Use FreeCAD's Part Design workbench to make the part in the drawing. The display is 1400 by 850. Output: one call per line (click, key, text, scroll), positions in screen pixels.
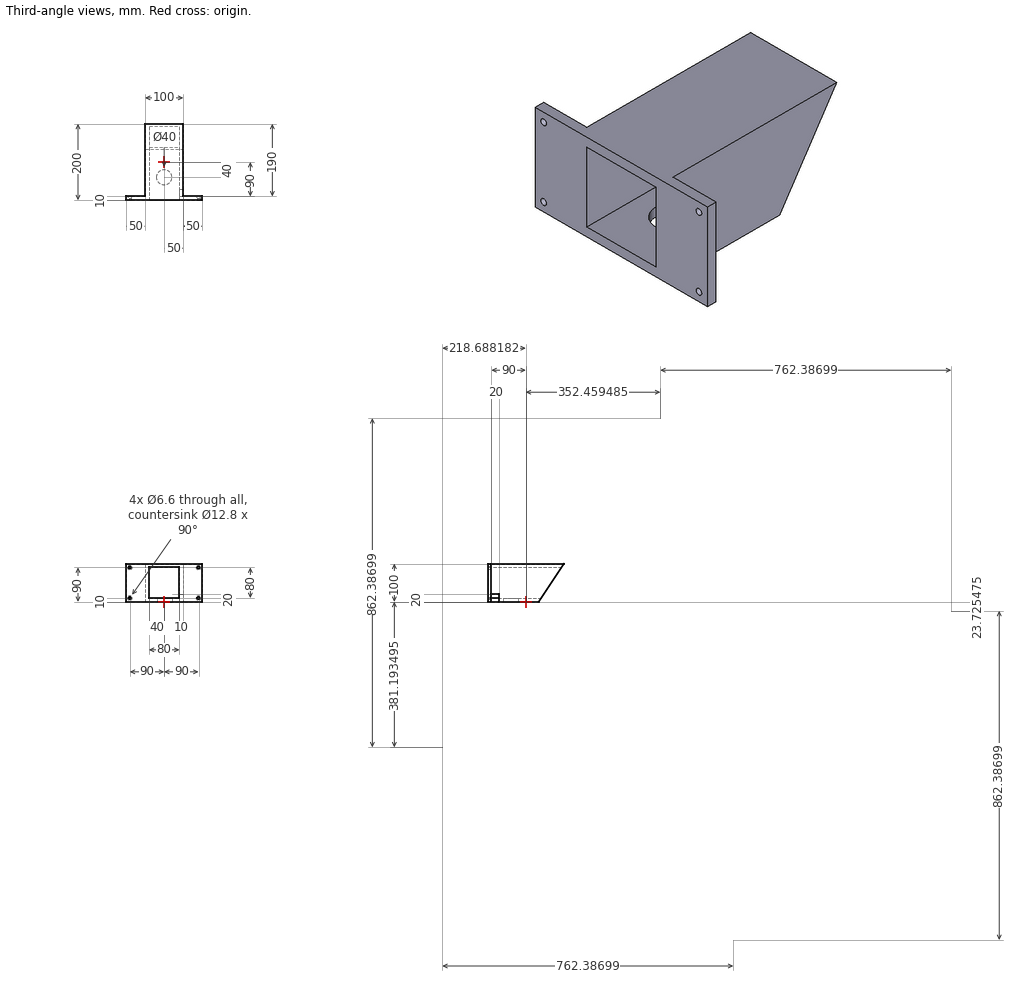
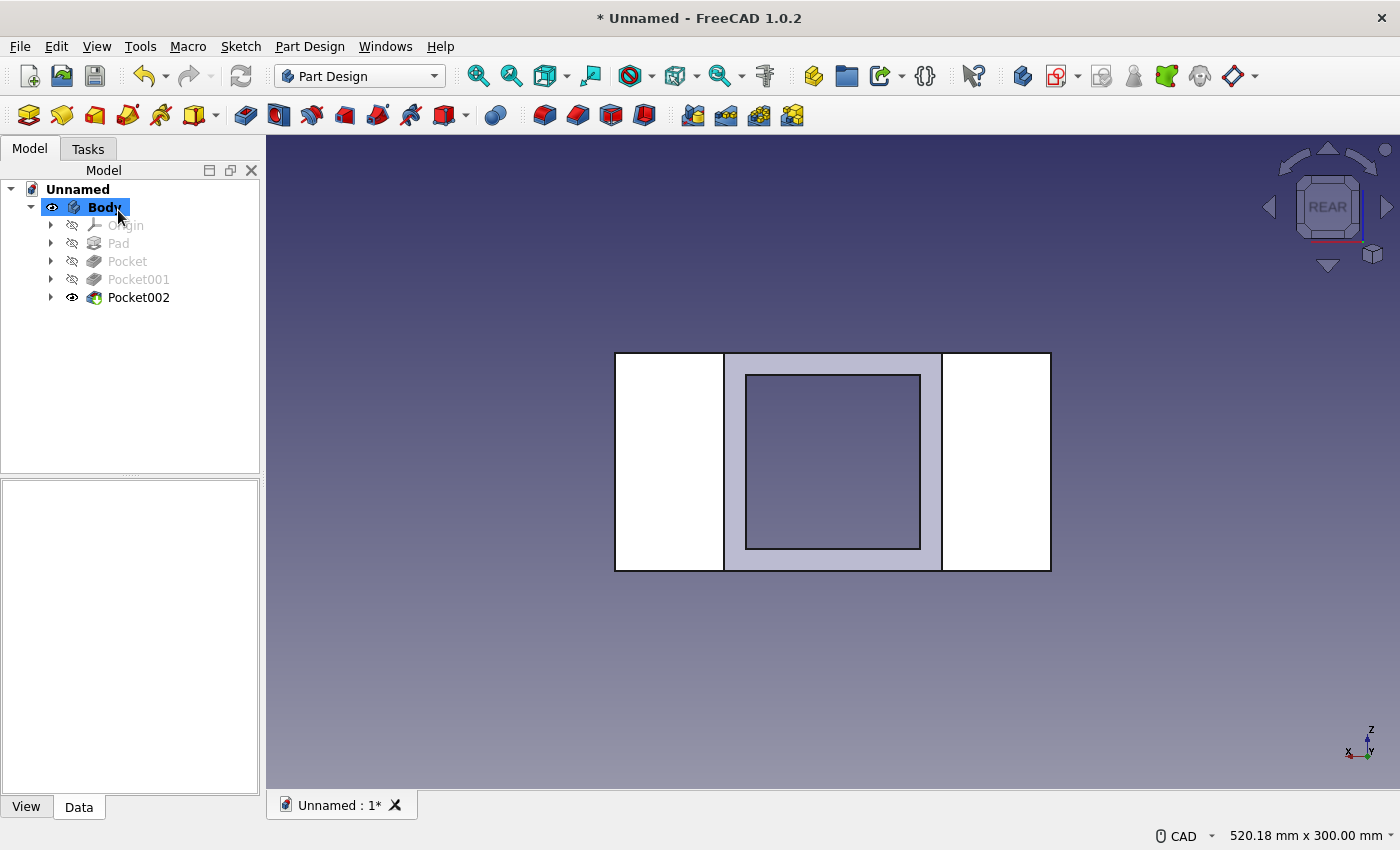
click(670, 430)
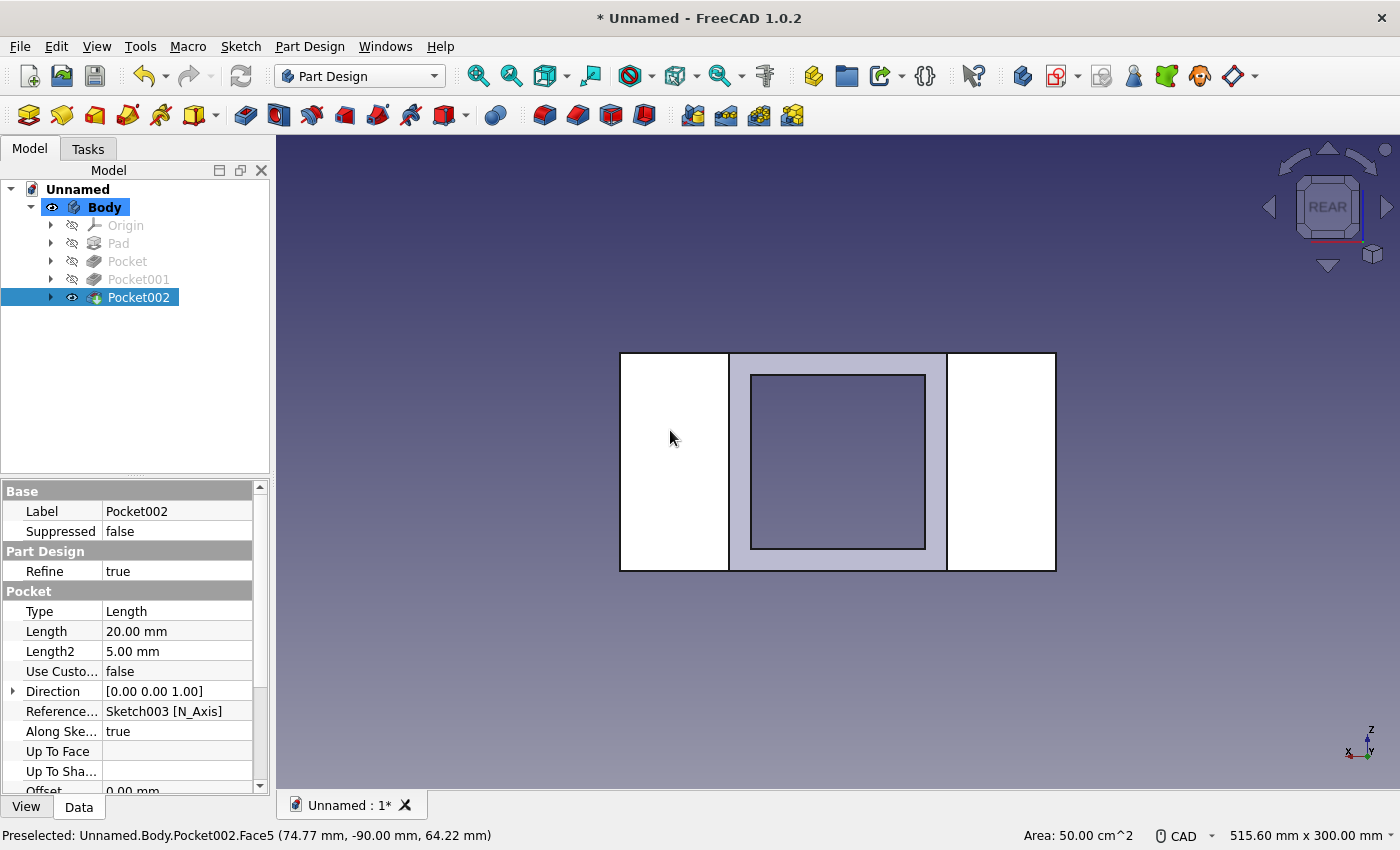
click(1056, 76)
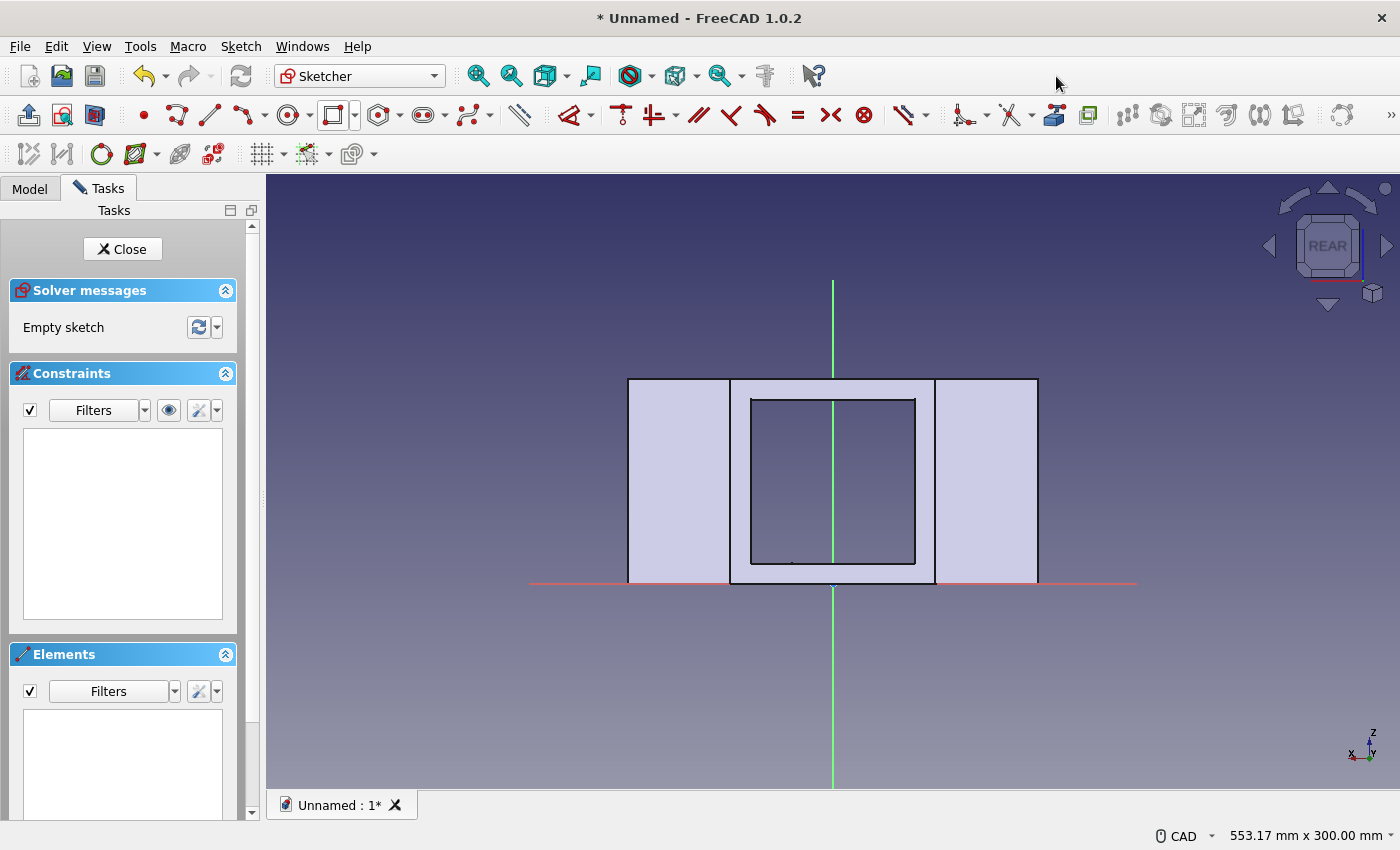
click(95, 116)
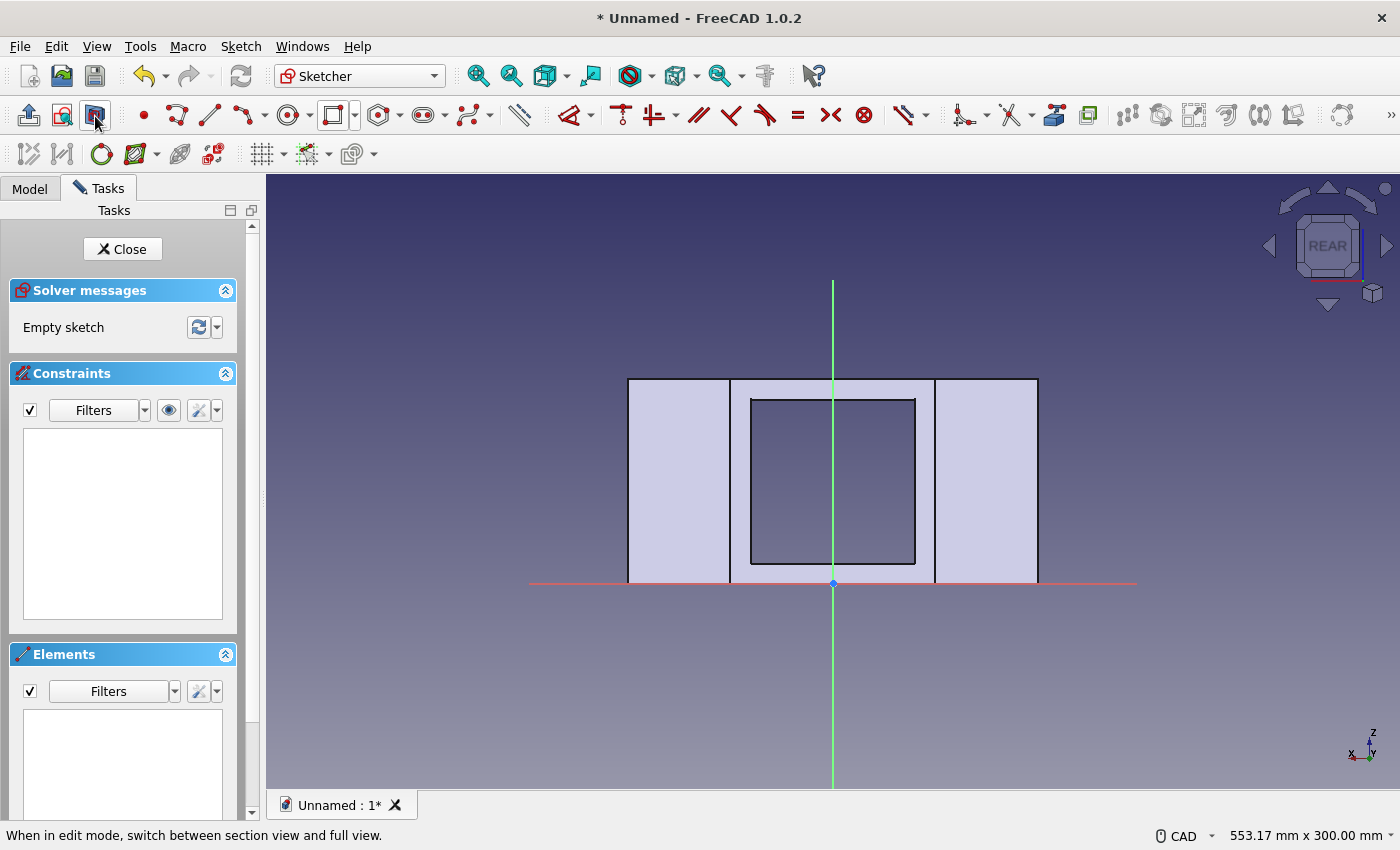
scroll(916, 497, up, 3)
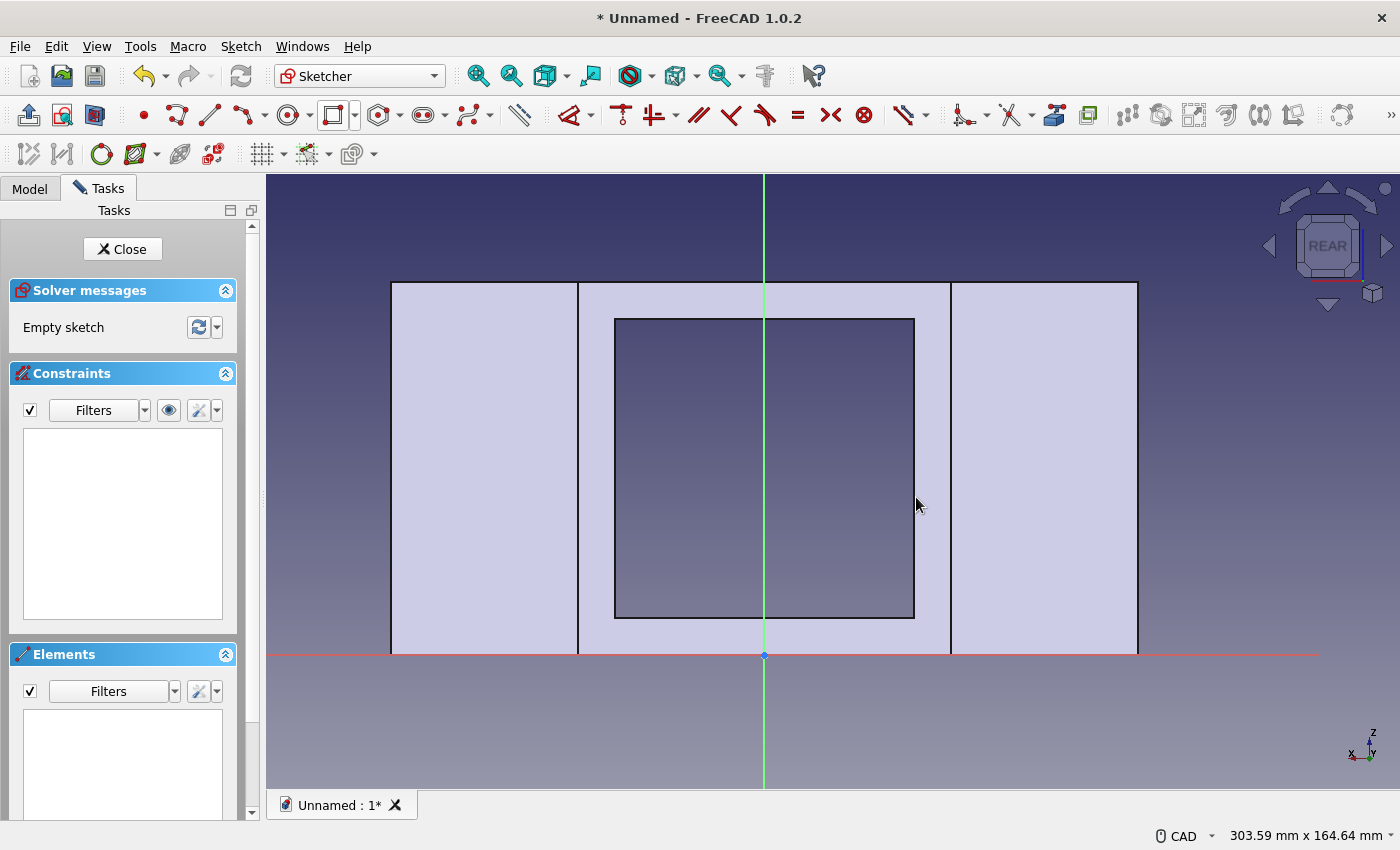
click(288, 116)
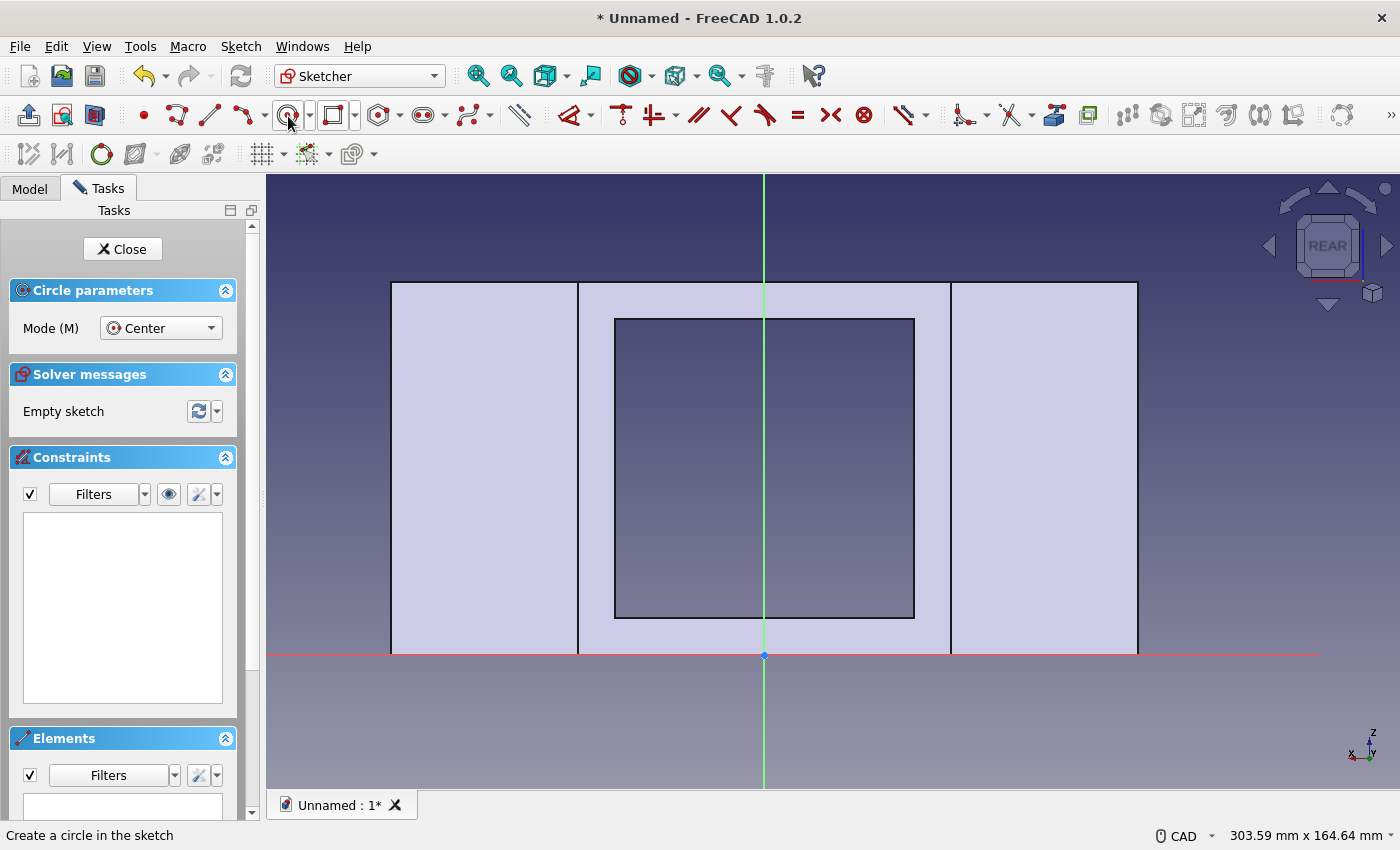
scroll(1100, 618, up, 4)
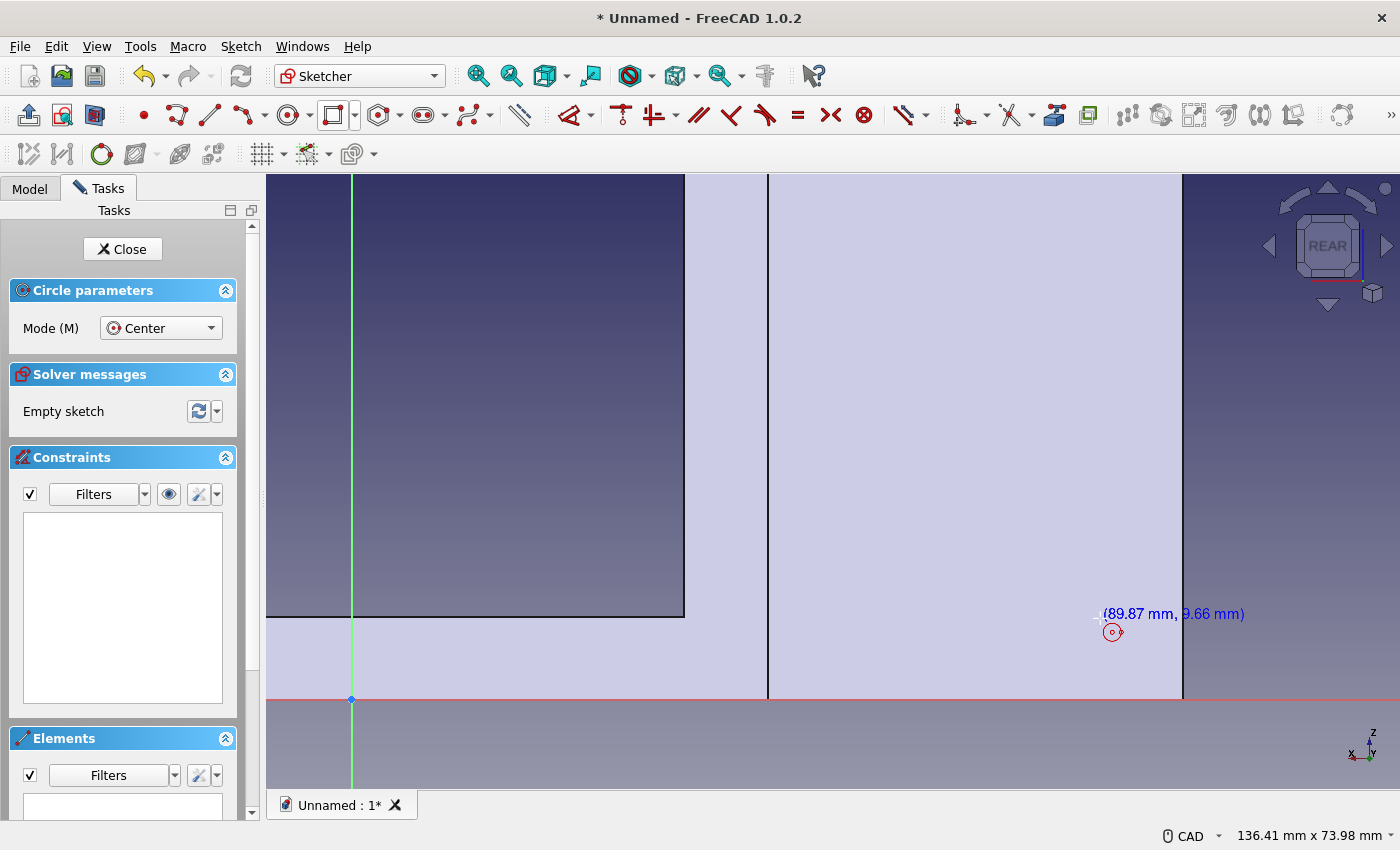
click(1100, 617)
move(1120, 597)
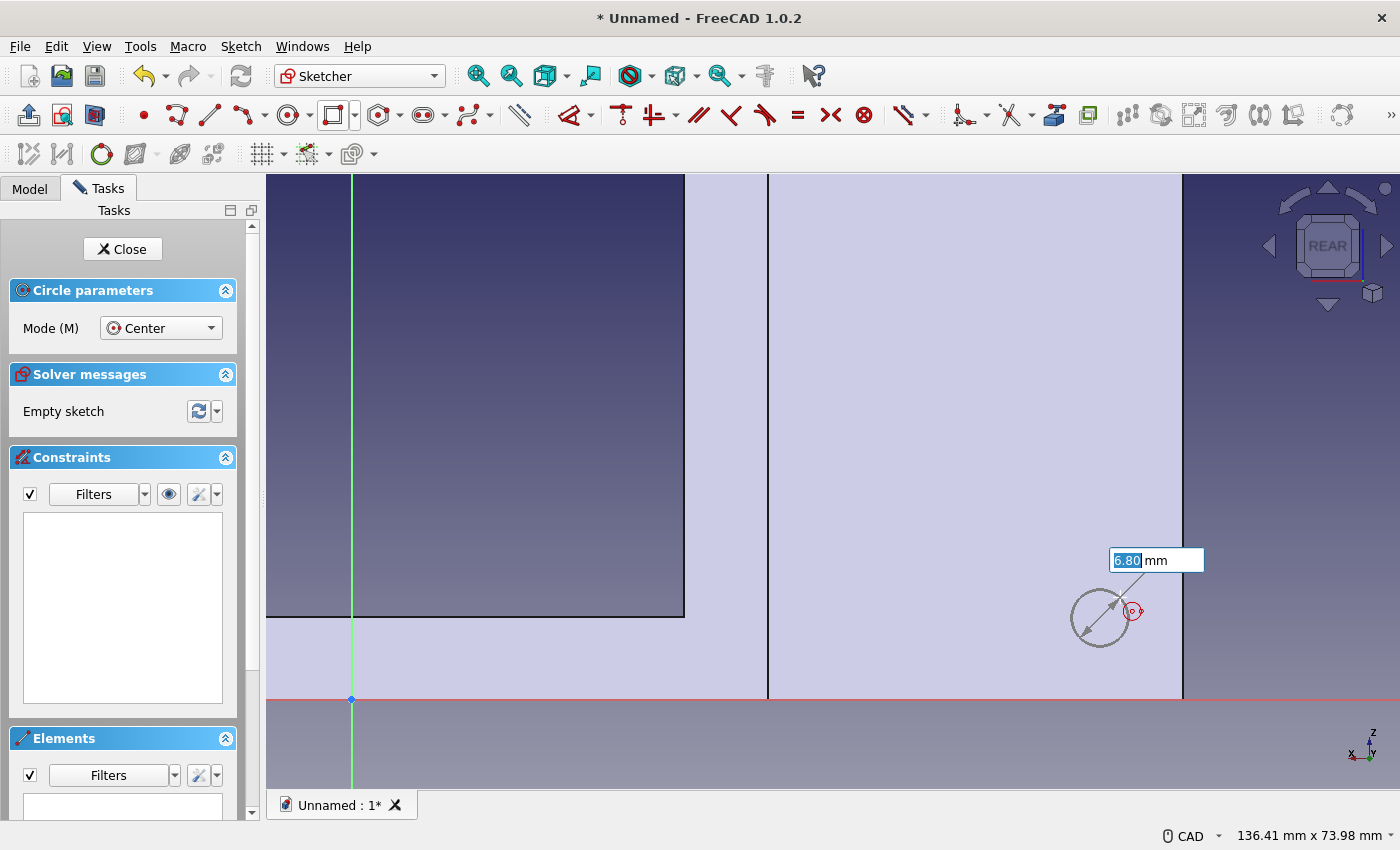
text(6.6)
key(Return)